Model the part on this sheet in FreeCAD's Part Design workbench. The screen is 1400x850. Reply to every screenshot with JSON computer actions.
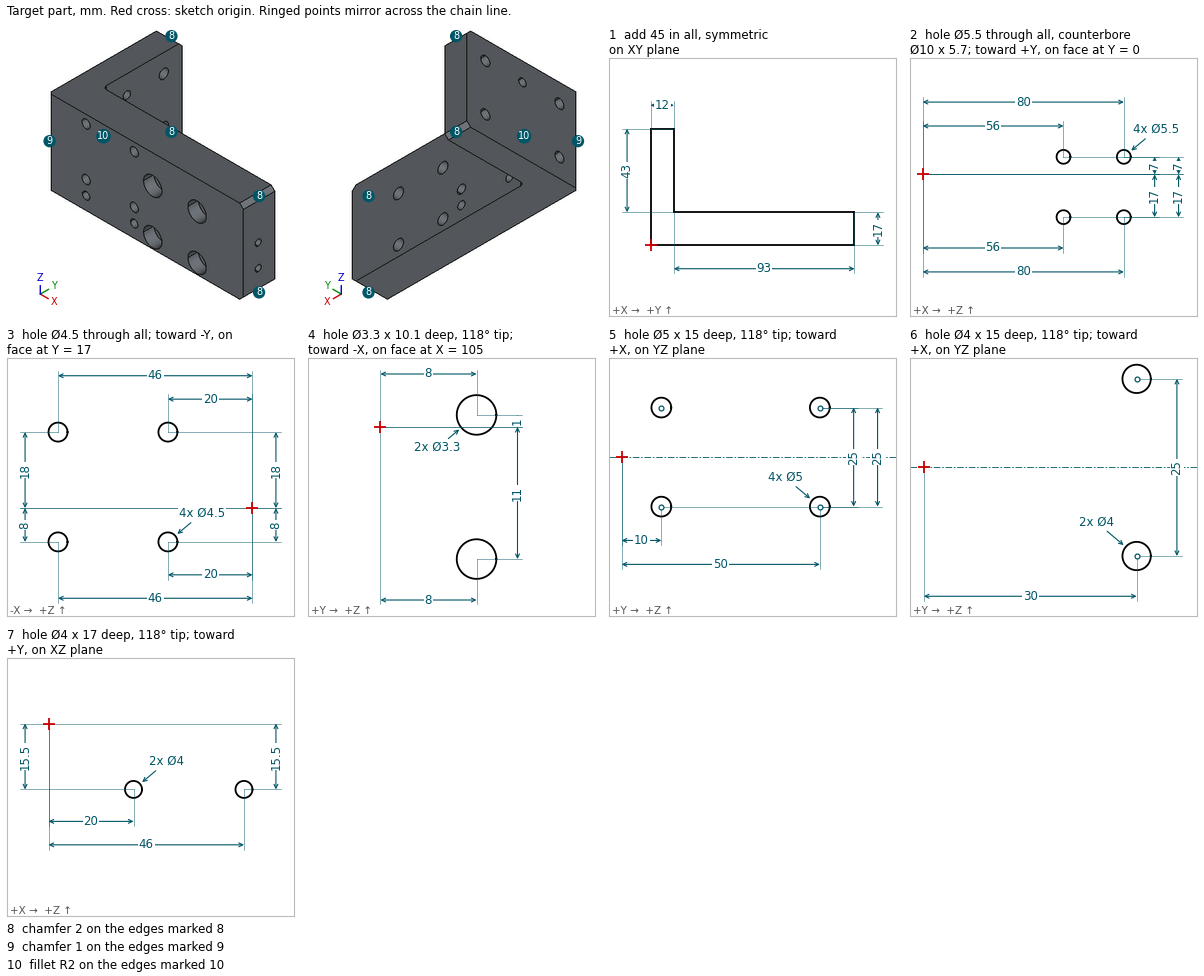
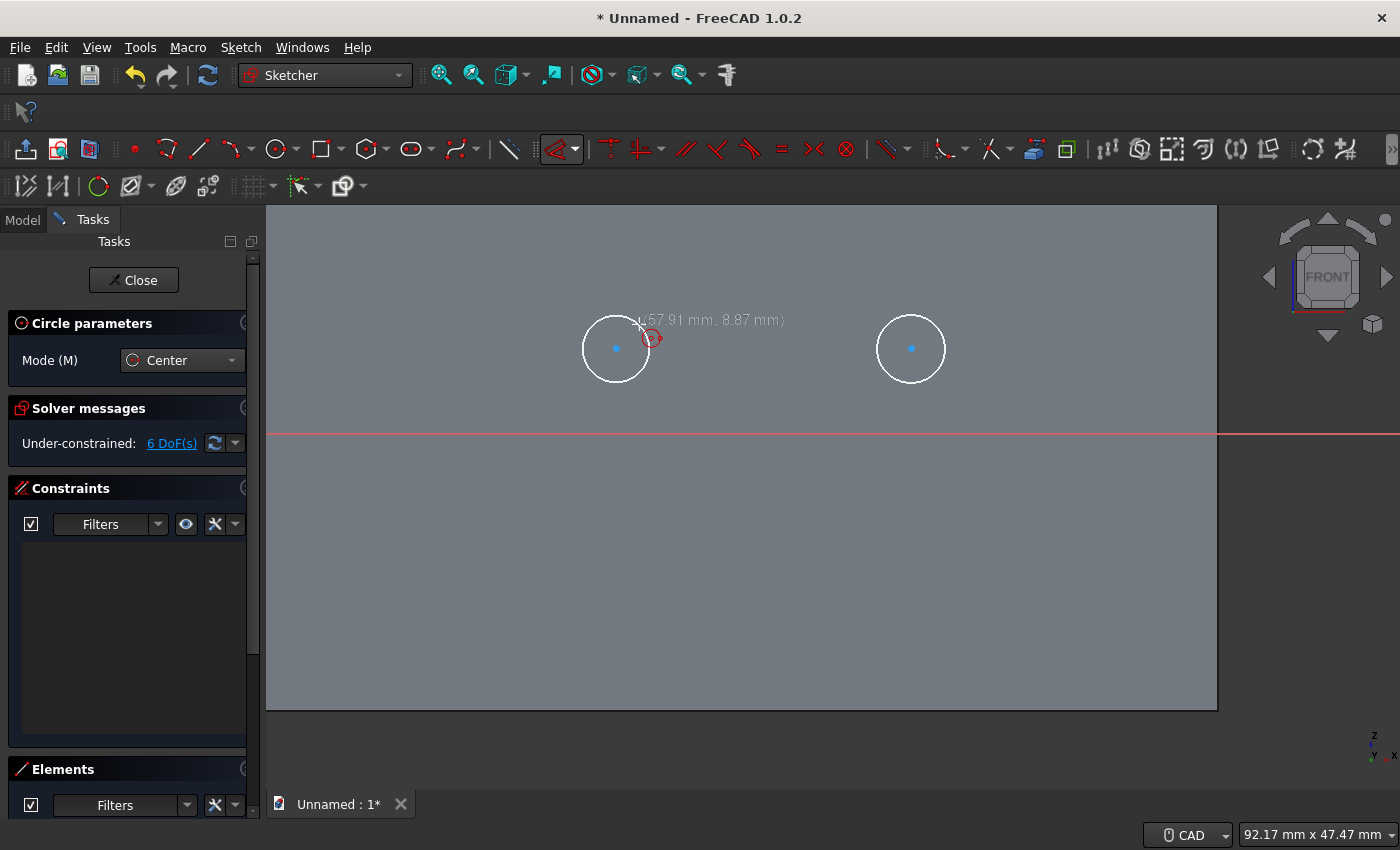
{"action": "left_click", "coordinate": [616, 643]}
{"action": "left_click", "coordinate": [639, 619]}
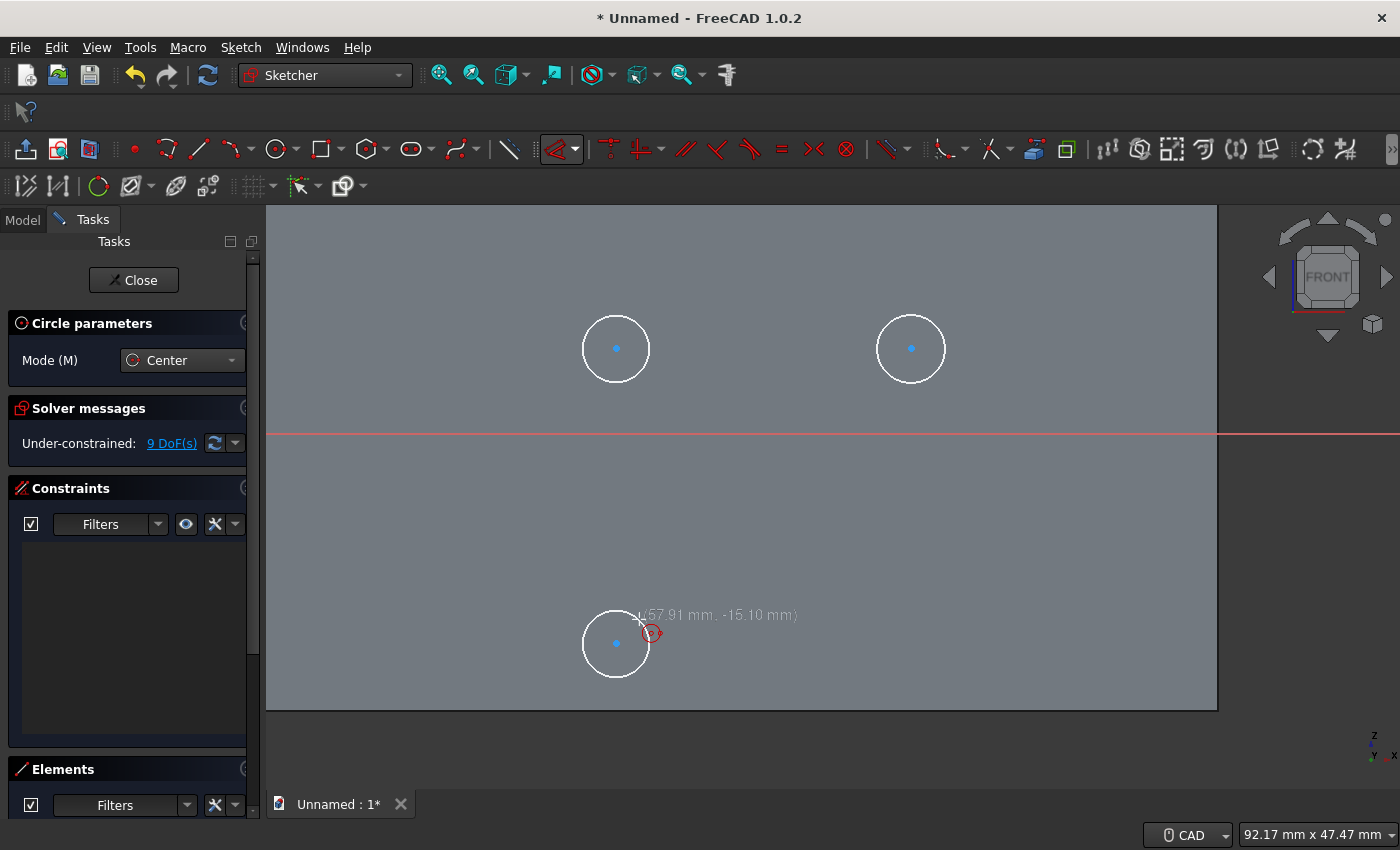
{"action": "left_click", "coordinate": [911, 643]}
{"action": "left_click", "coordinate": [935, 619]}
{"action": "key", "text": "Escape"}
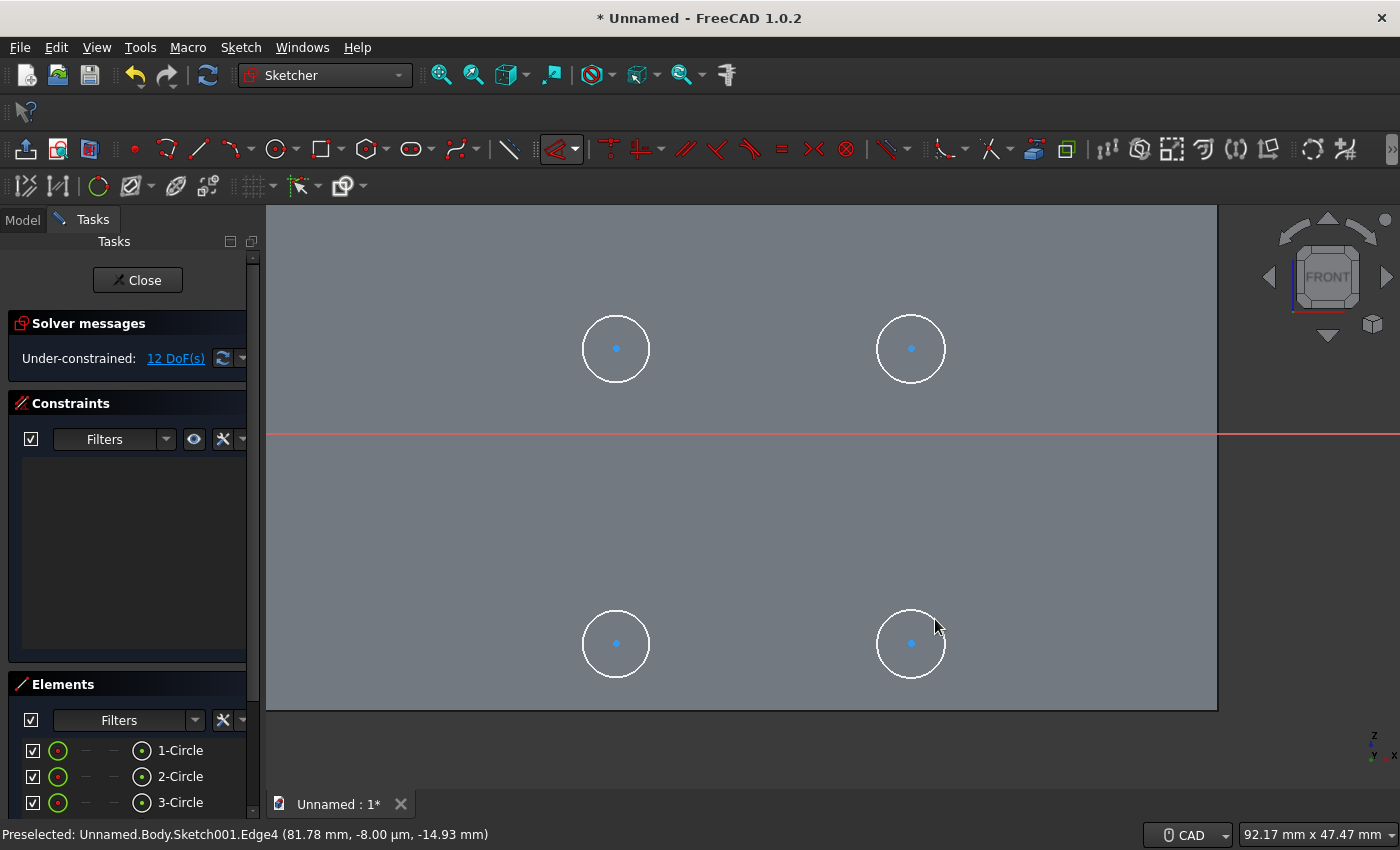
{"action": "left_click", "coordinate": [935, 325]}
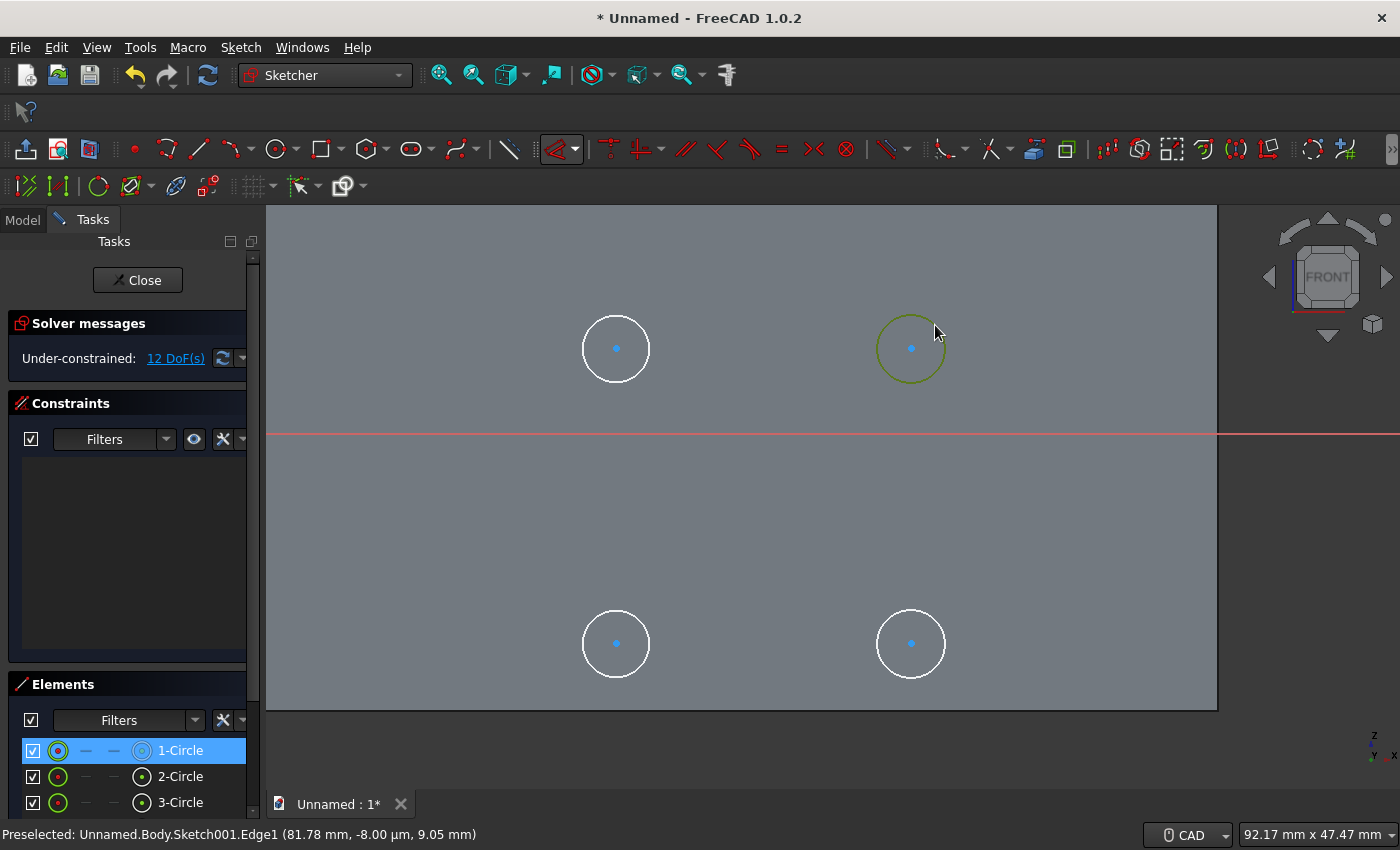
{"action": "left_click", "coordinate": [639, 325]}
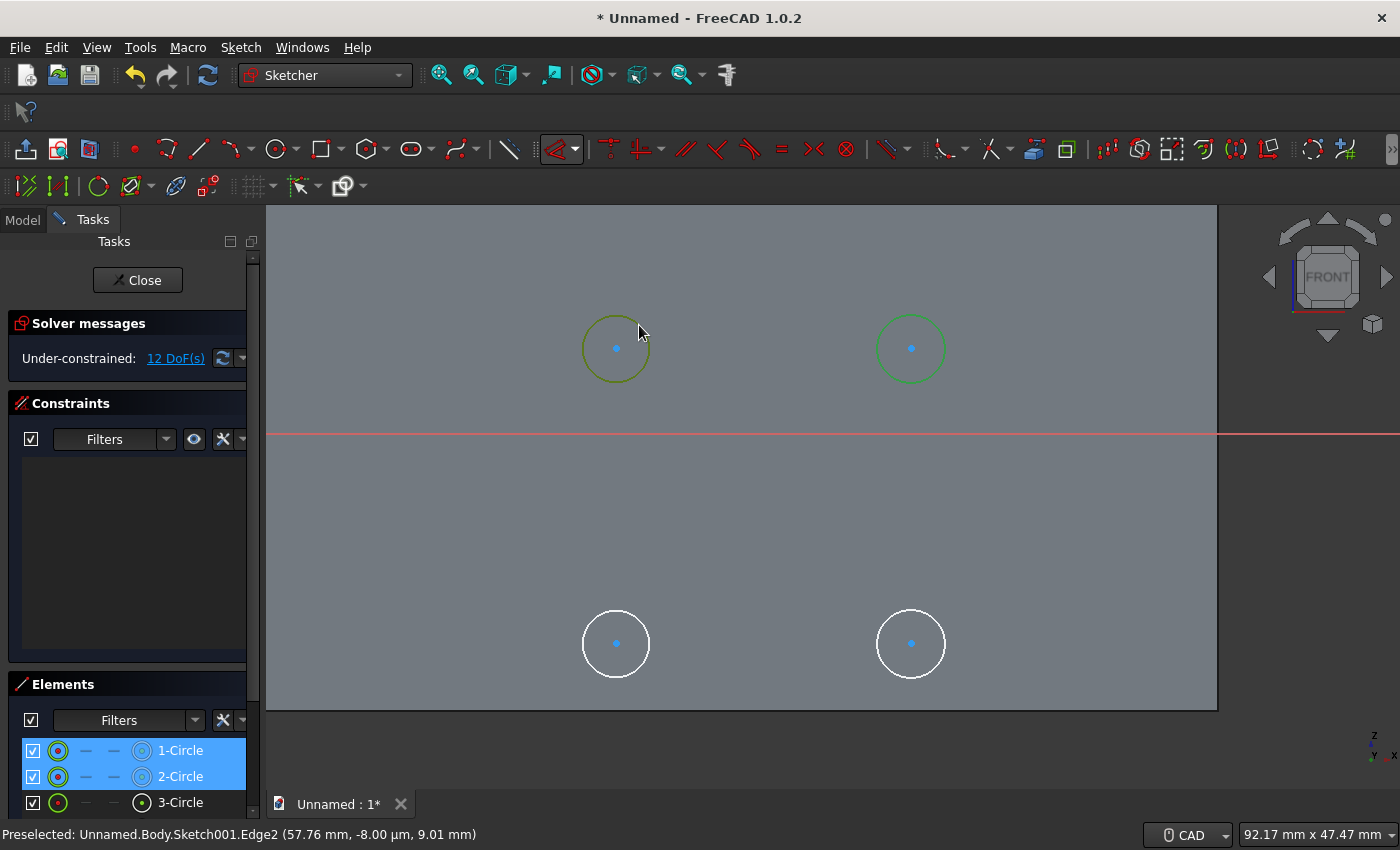
{"action": "left_click", "coordinate": [639, 620]}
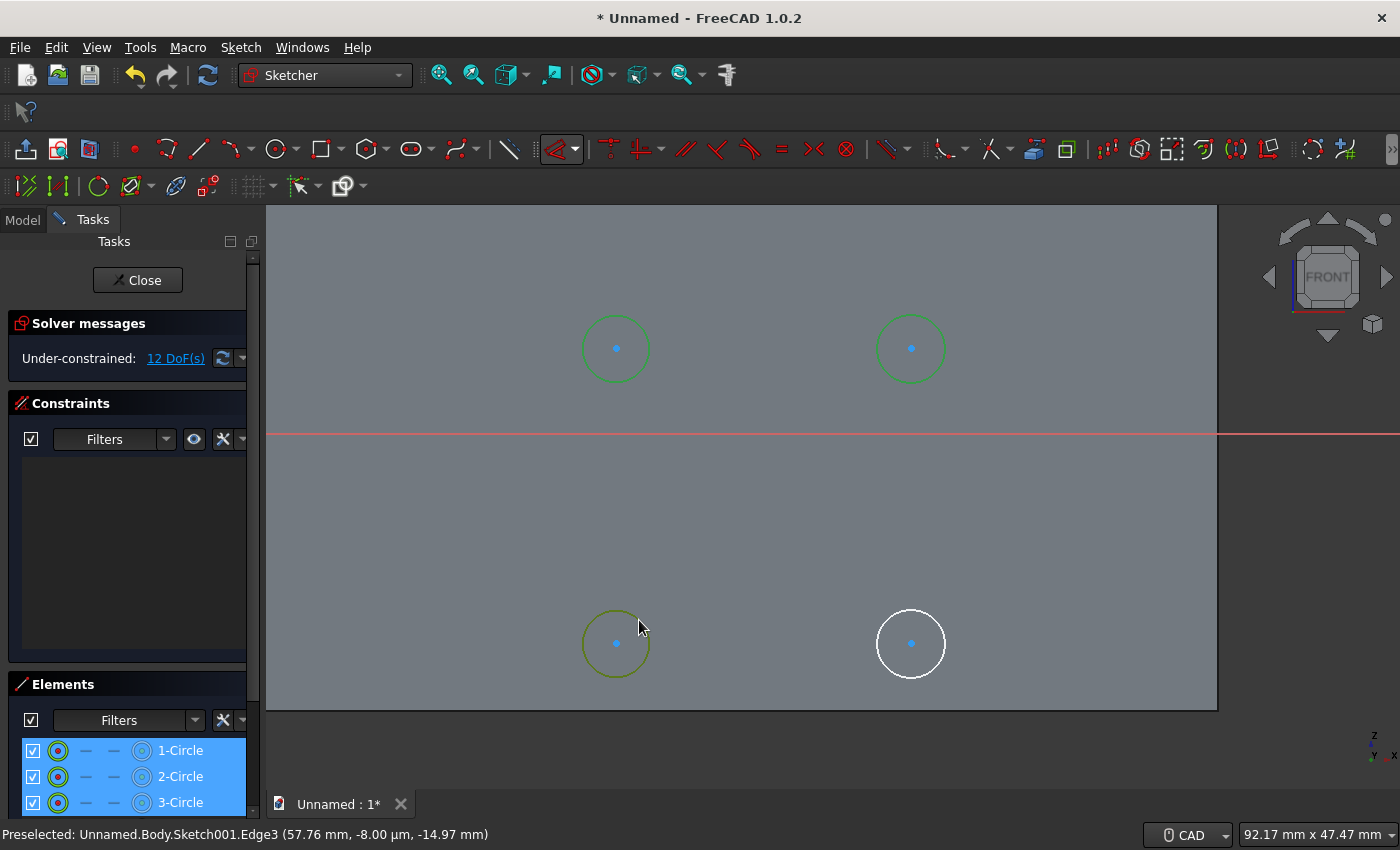
{"action": "left_click", "coordinate": [935, 620]}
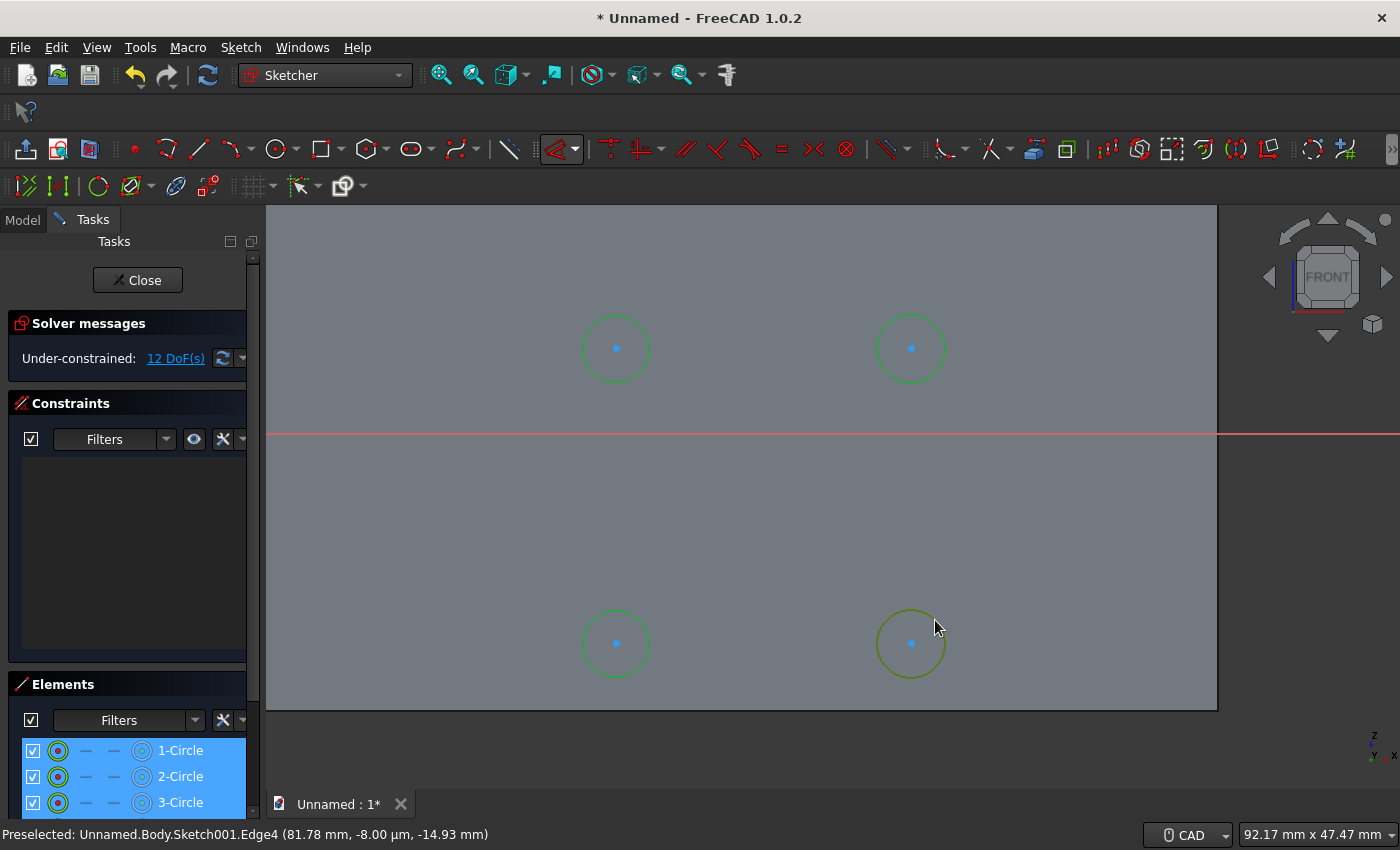
{"action": "left_click", "coordinate": [782, 150]}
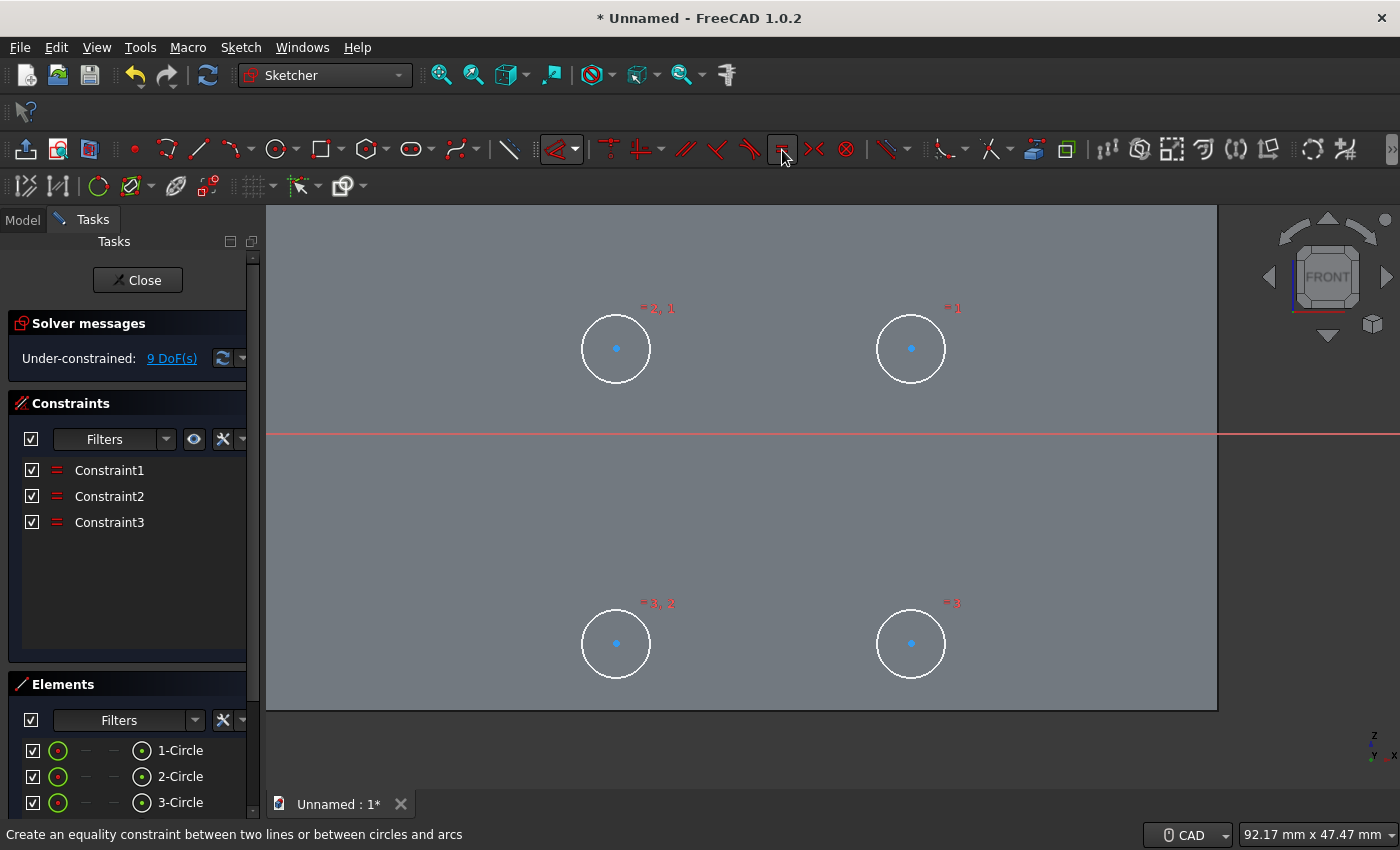
{"action": "left_click", "coordinate": [935, 325]}